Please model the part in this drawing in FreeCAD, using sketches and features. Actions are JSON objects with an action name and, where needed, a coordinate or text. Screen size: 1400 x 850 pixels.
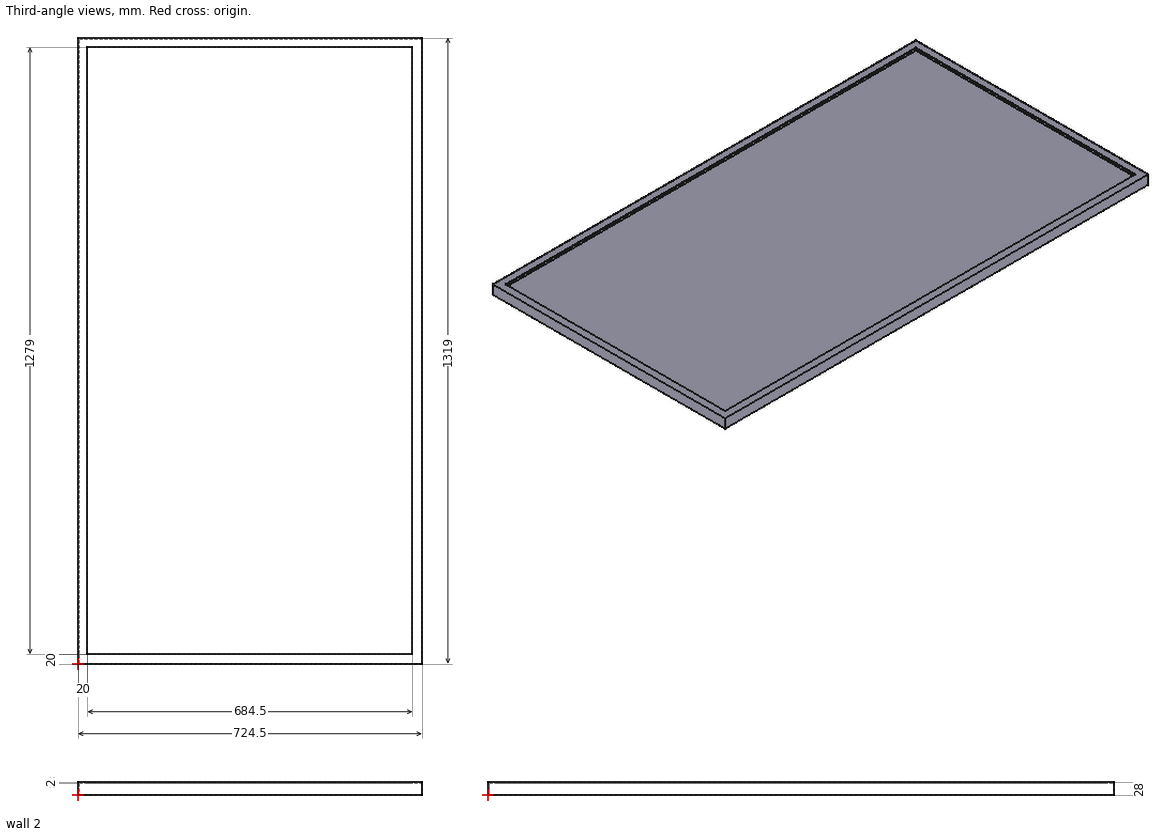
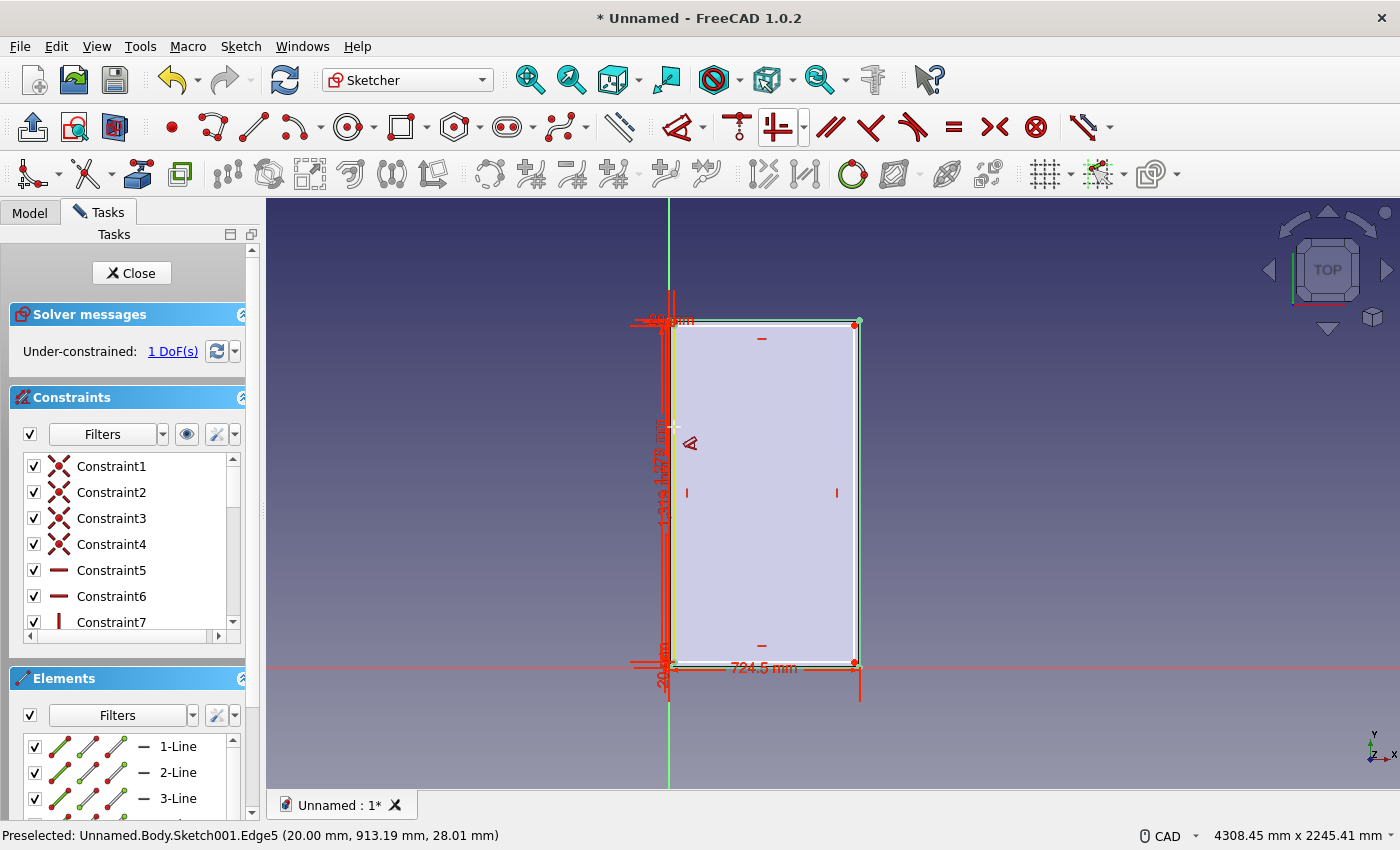
{"action": "scroll", "coordinate": [728, 662], "scroll_direction": "up", "scroll_amount": 5}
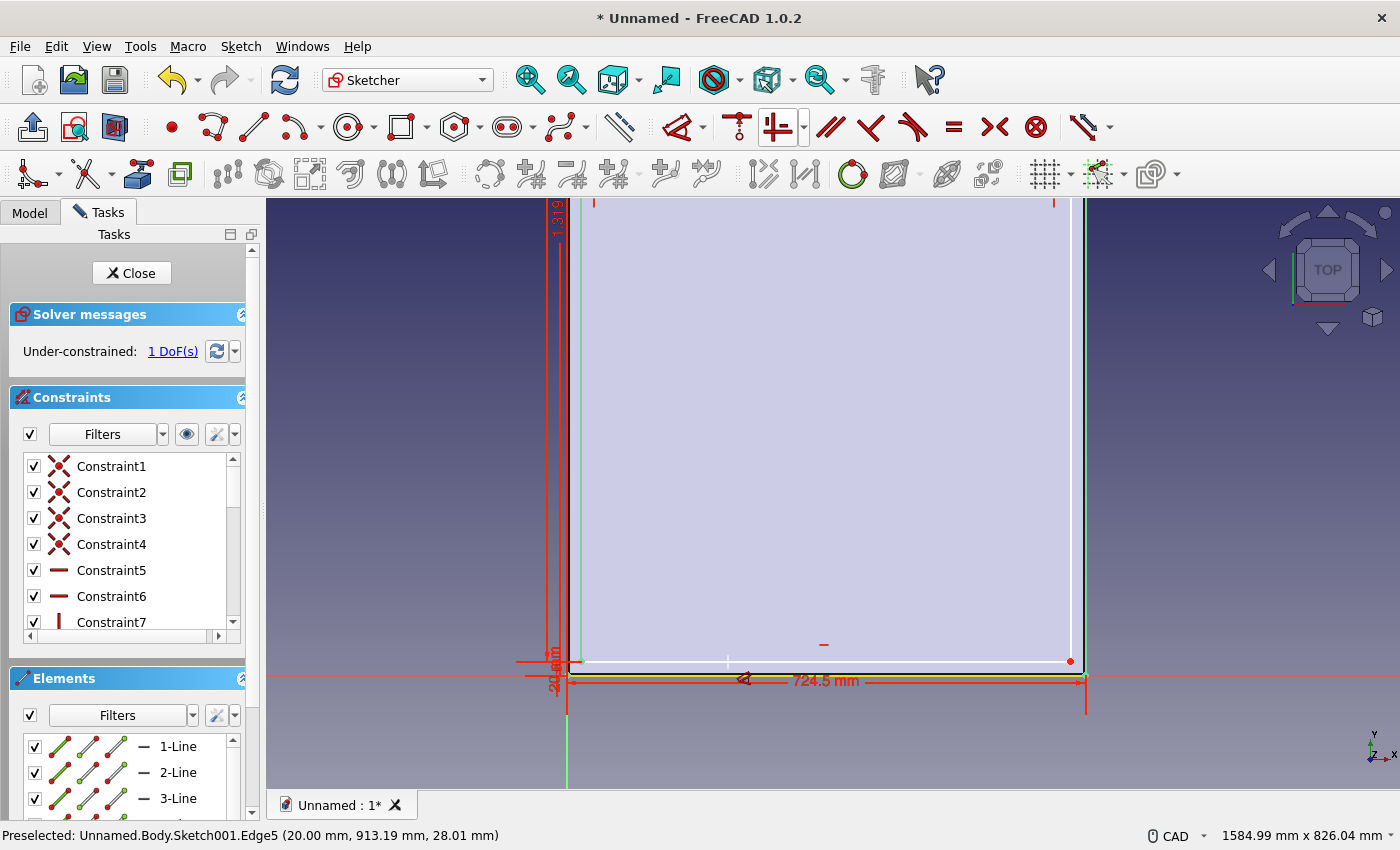
{"action": "left_click", "coordinate": [728, 662]}
{"action": "left_click", "coordinate": [826, 696]}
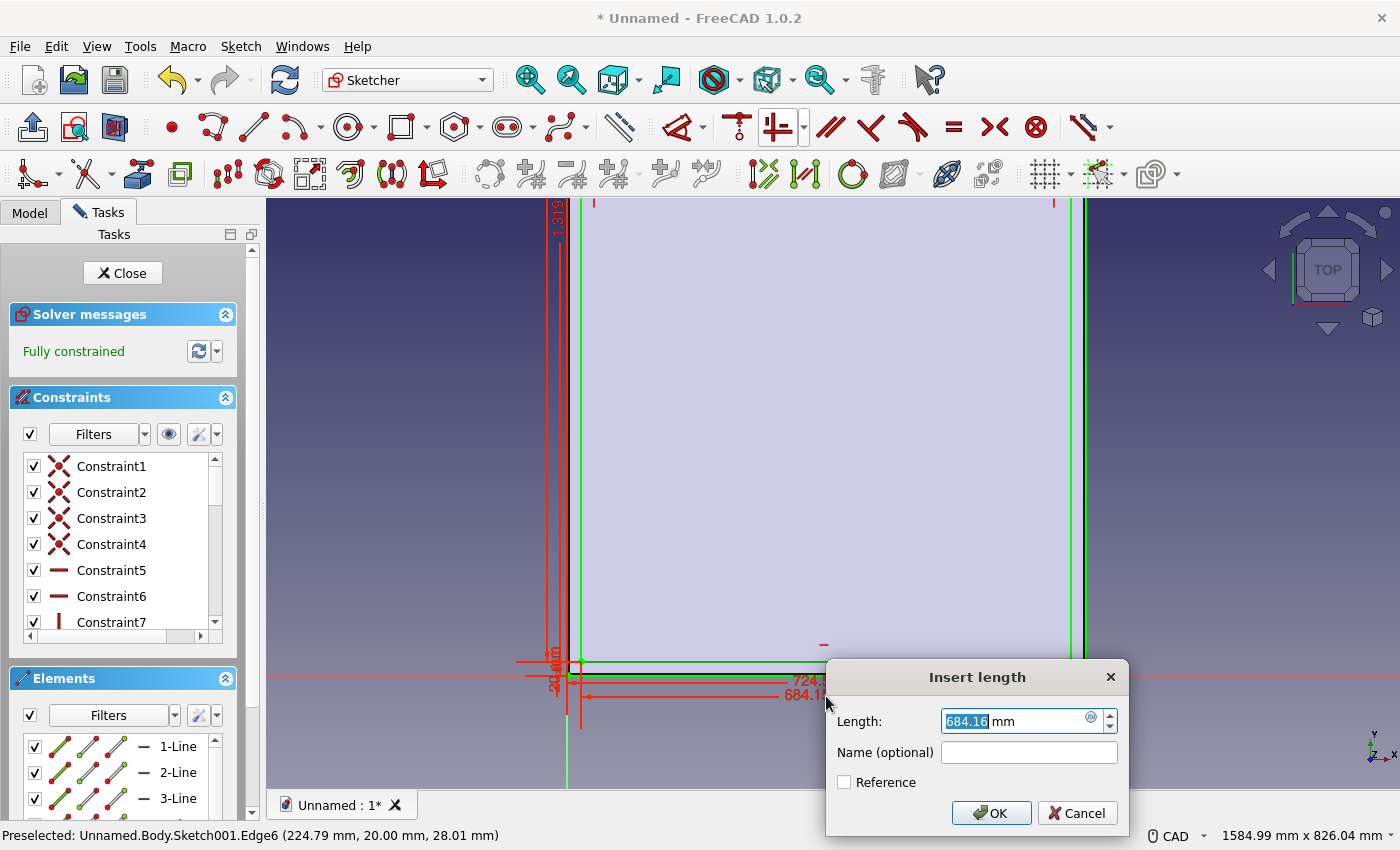
{"action": "type", "text": "684.5"}
{"action": "key", "text": "Return"}
{"action": "key", "text": "Escape"}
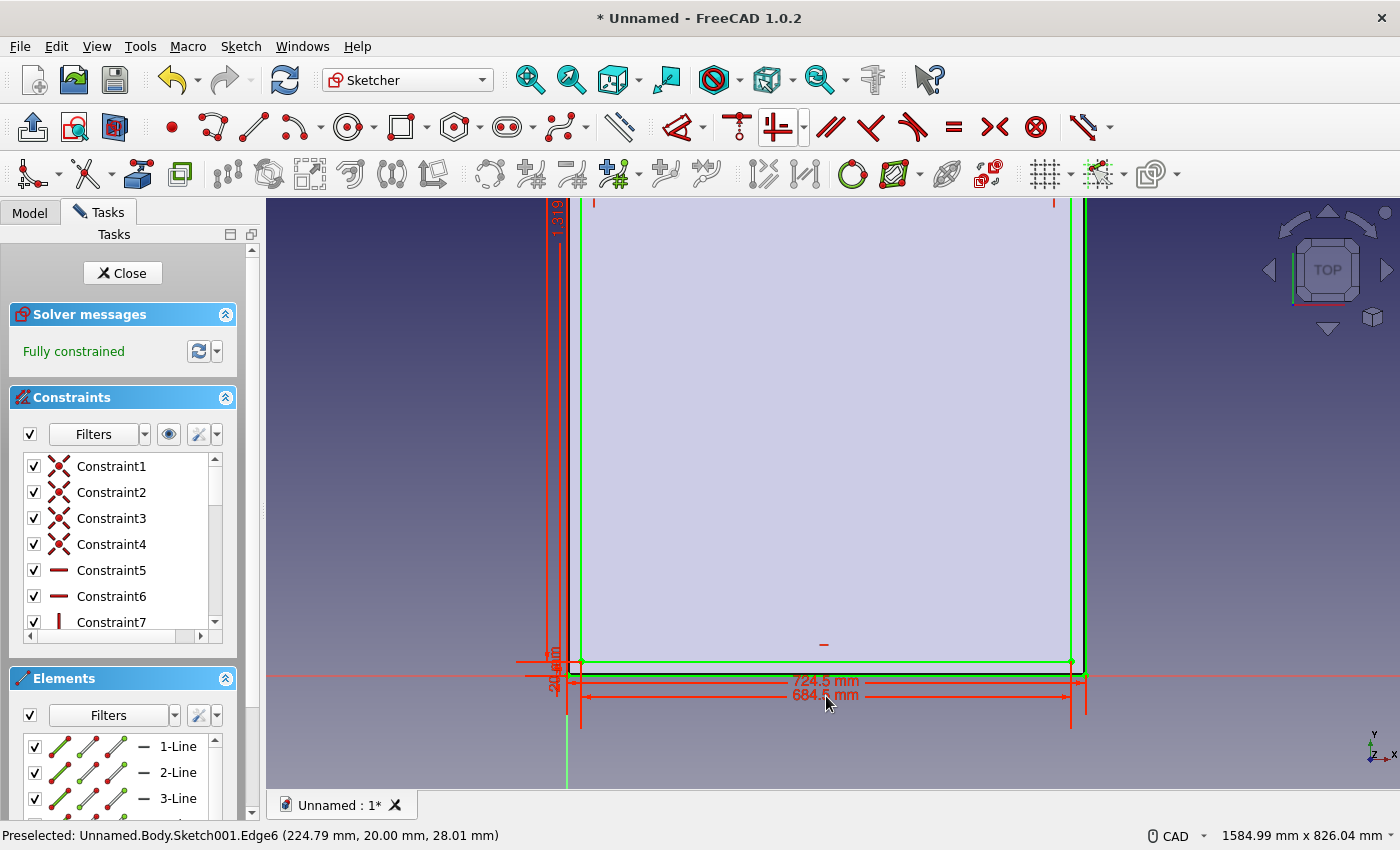
{"action": "left_click", "coordinate": [123, 273]}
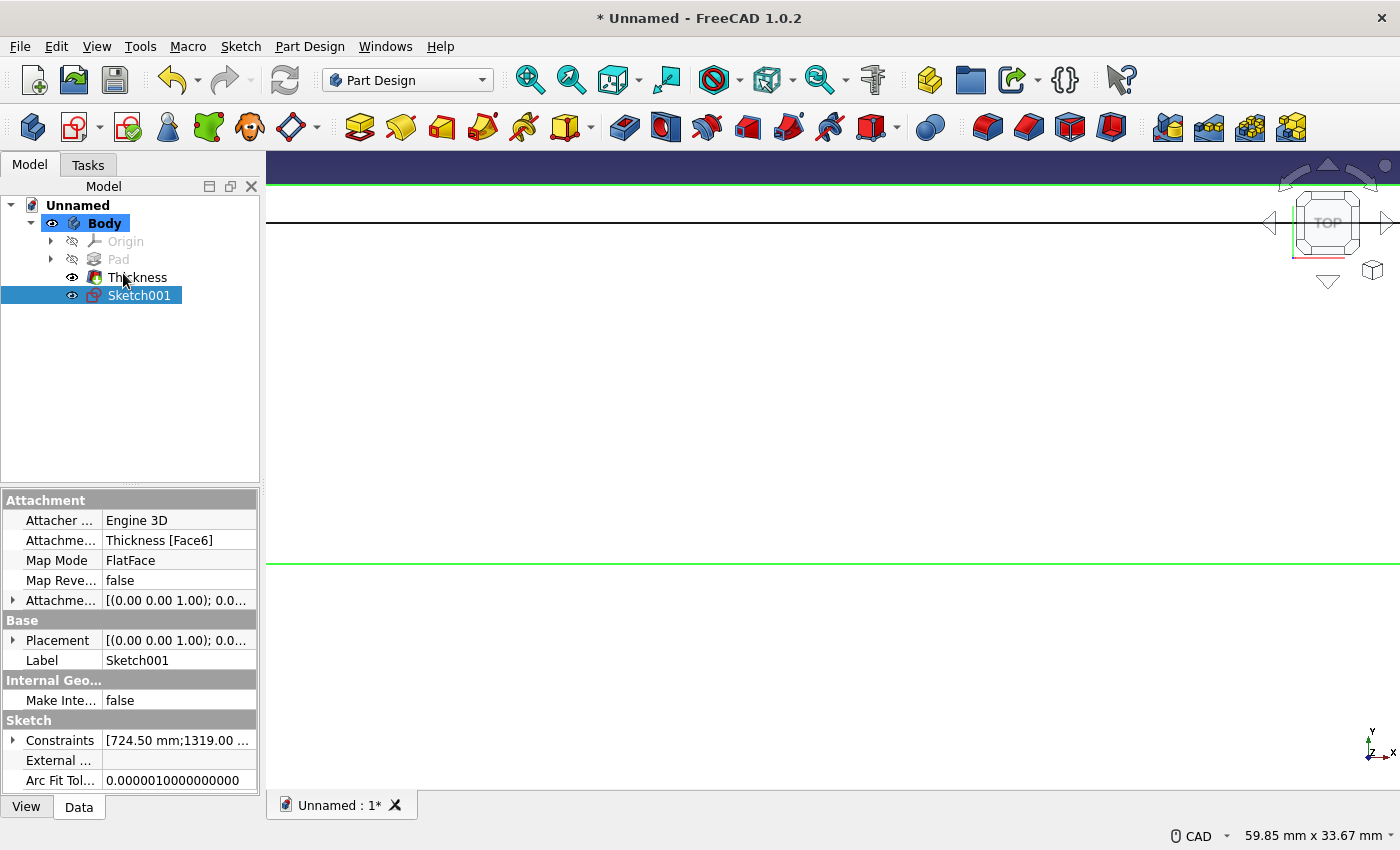
{"action": "left_click", "coordinate": [360, 128]}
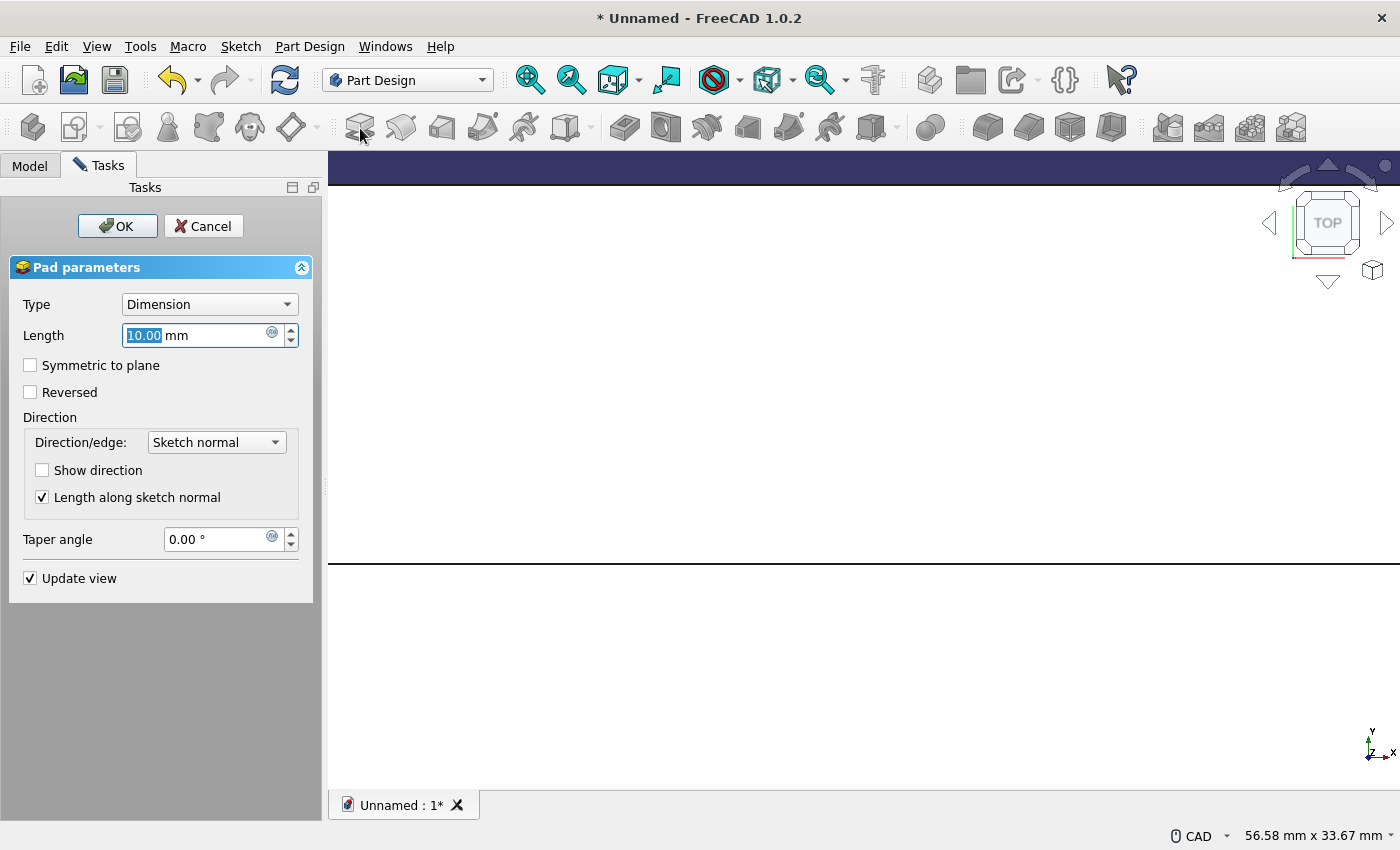
{"action": "type", "text": "2"}
{"action": "key", "text": "Tab"}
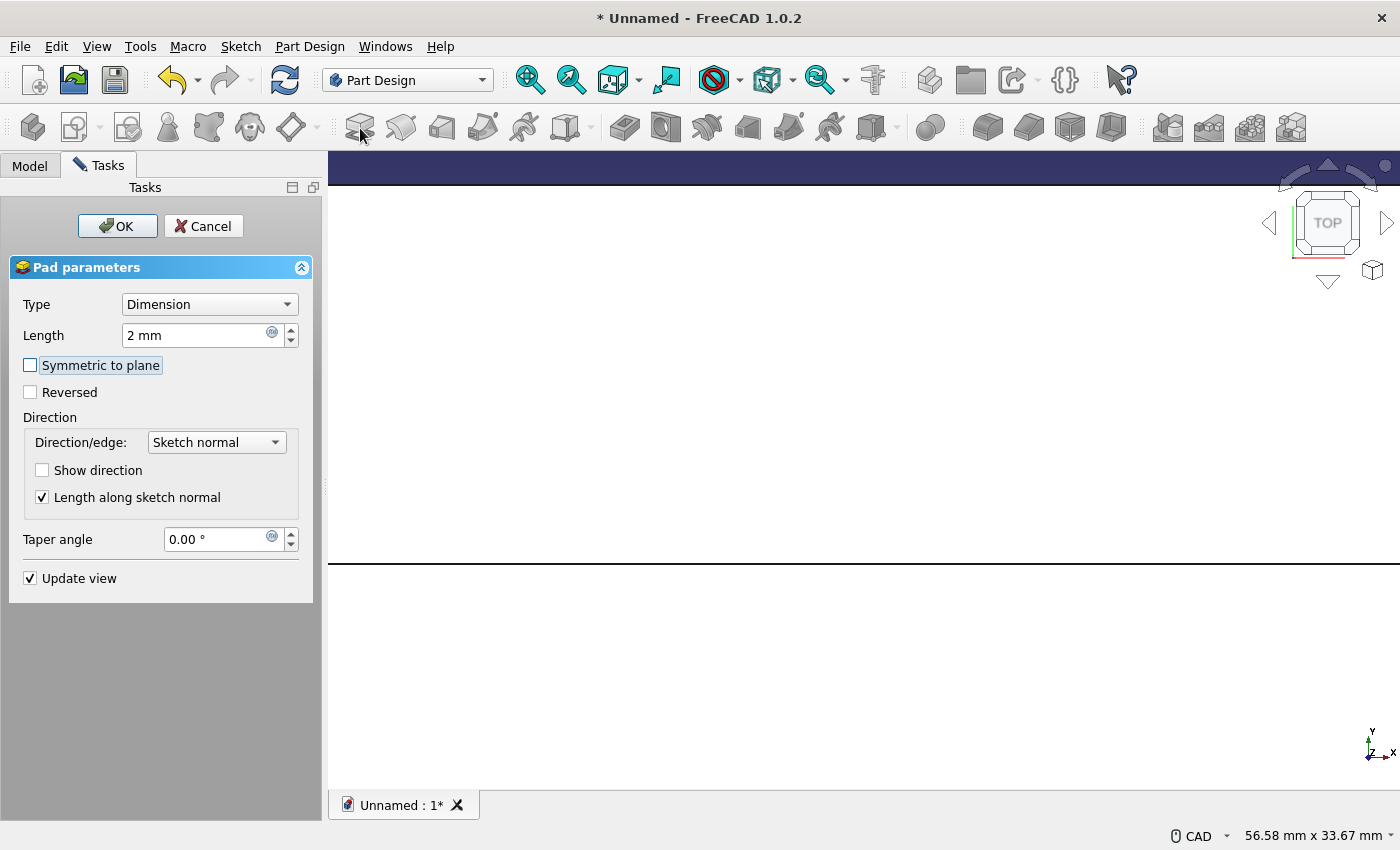
{"action": "left_click", "coordinate": [31, 392]}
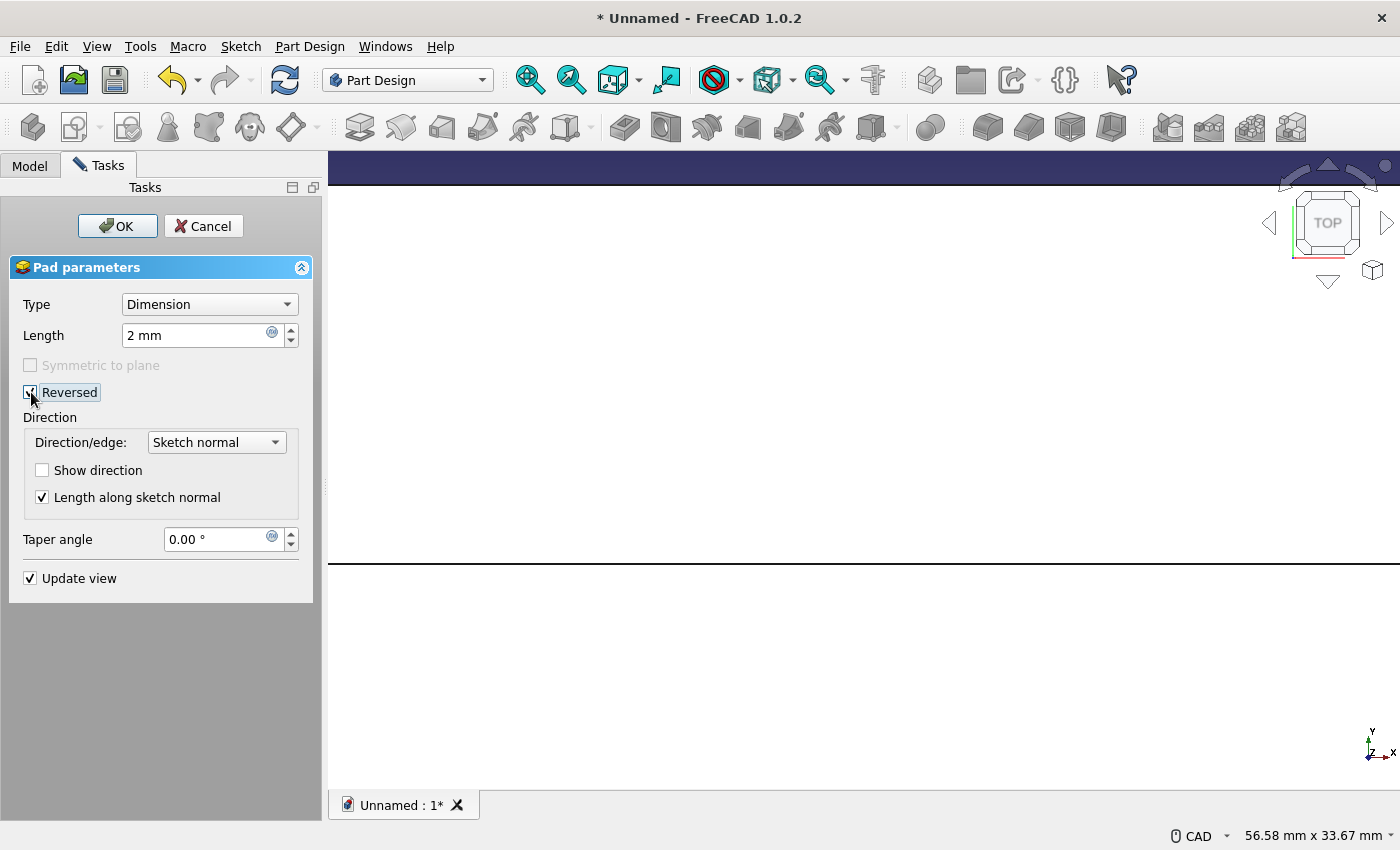
{"action": "left_click", "coordinate": [118, 226]}